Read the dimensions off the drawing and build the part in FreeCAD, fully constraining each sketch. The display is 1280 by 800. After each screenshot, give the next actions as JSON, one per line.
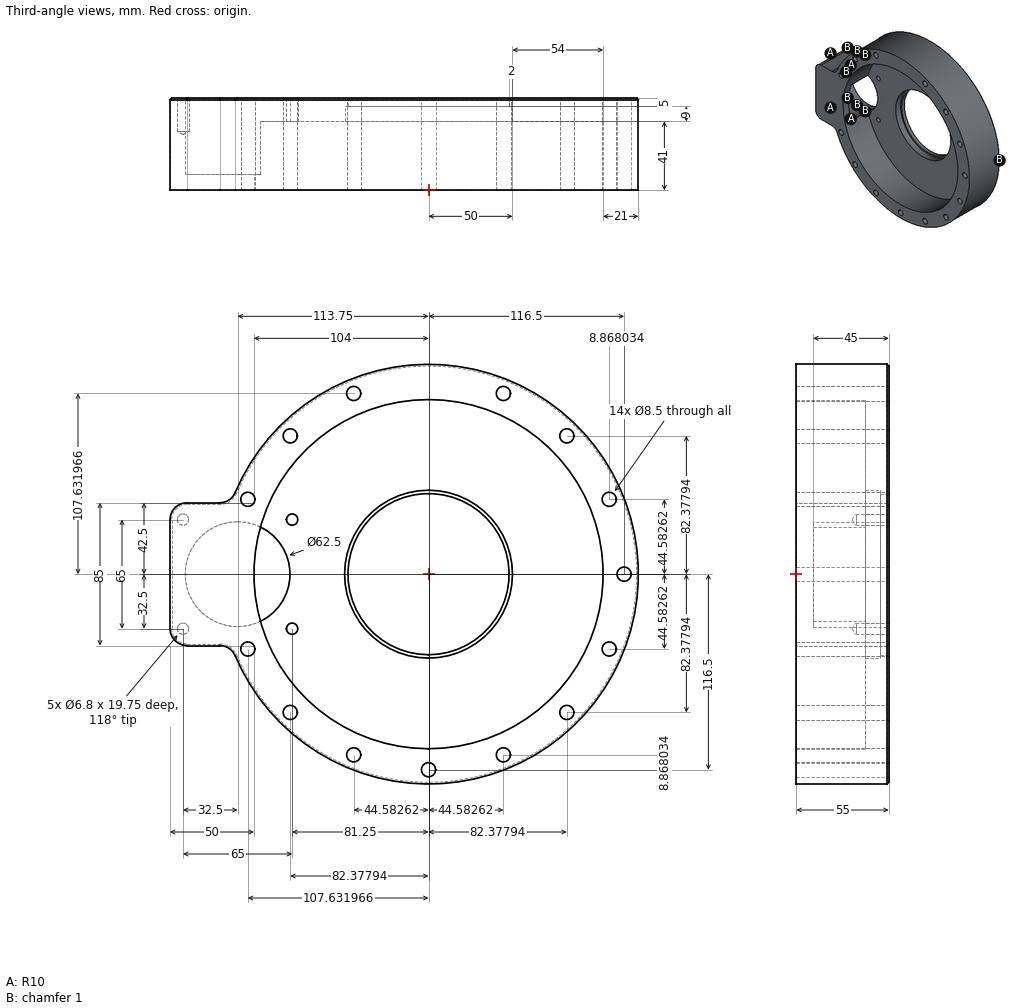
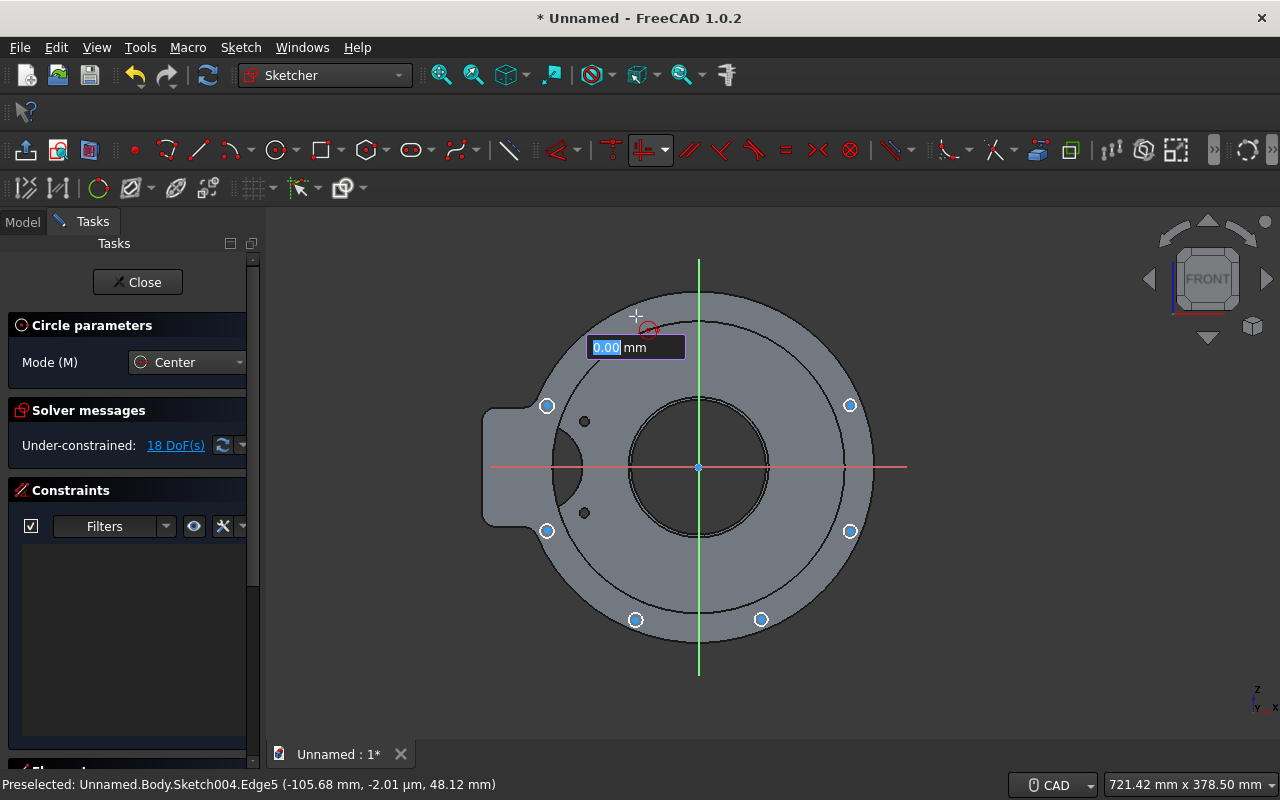
{"action": "scroll", "coordinate": [640, 312], "scroll_direction": "up", "scroll_amount": 5}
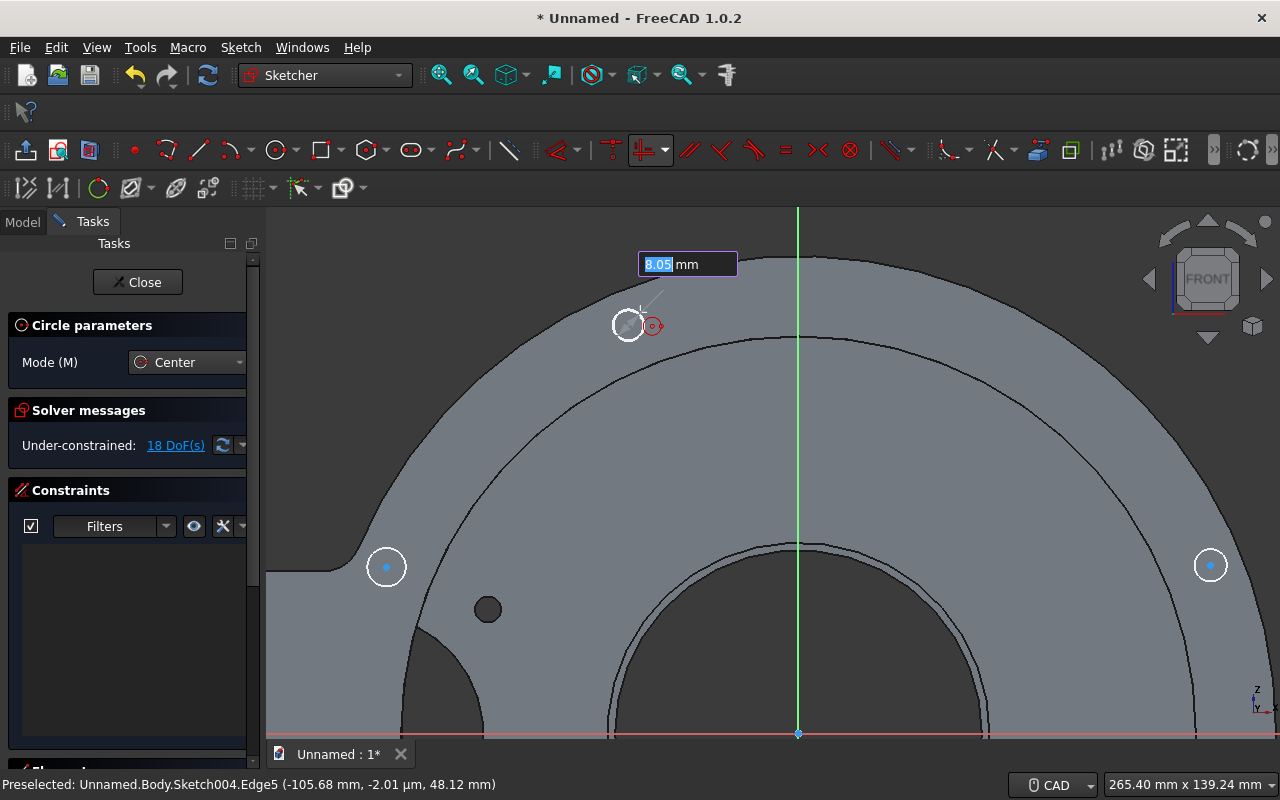
{"action": "left_click", "coordinate": [640, 311]}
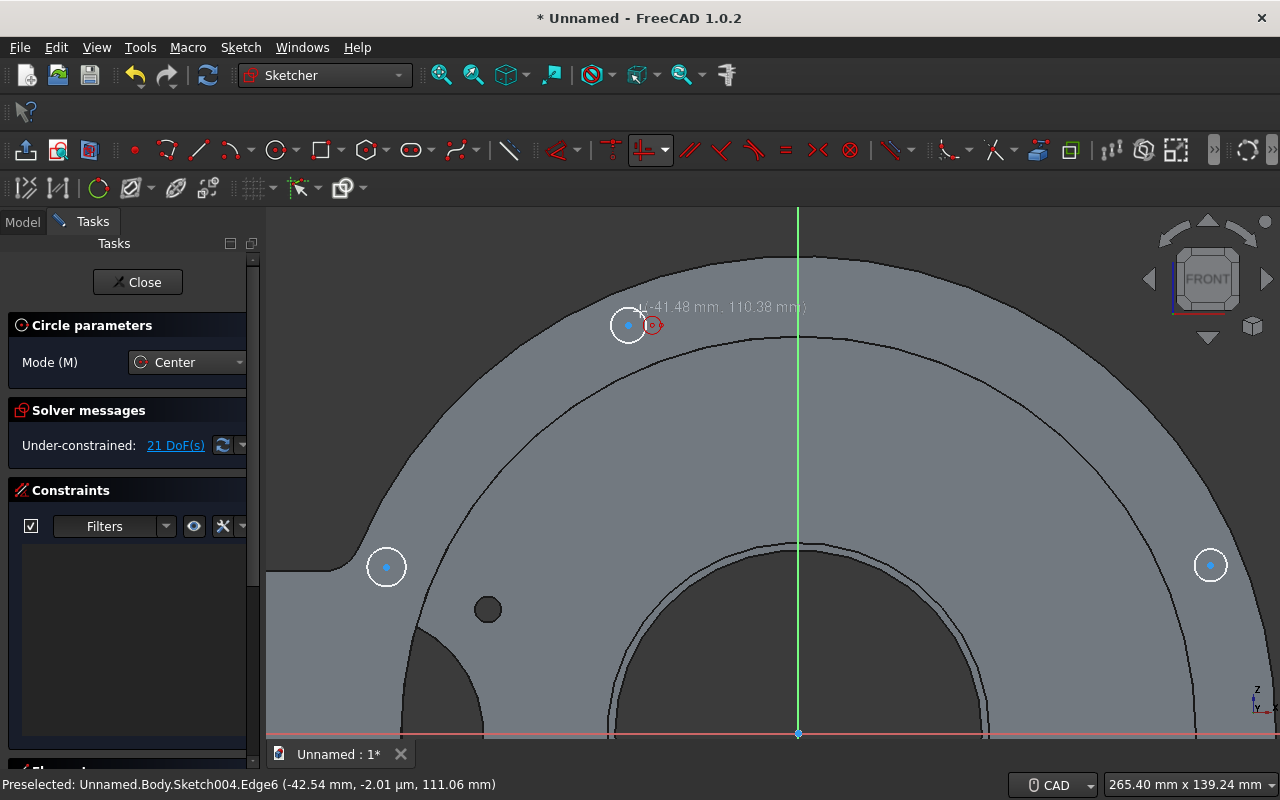
{"action": "scroll", "coordinate": [969, 323], "scroll_direction": "up", "scroll_amount": 2}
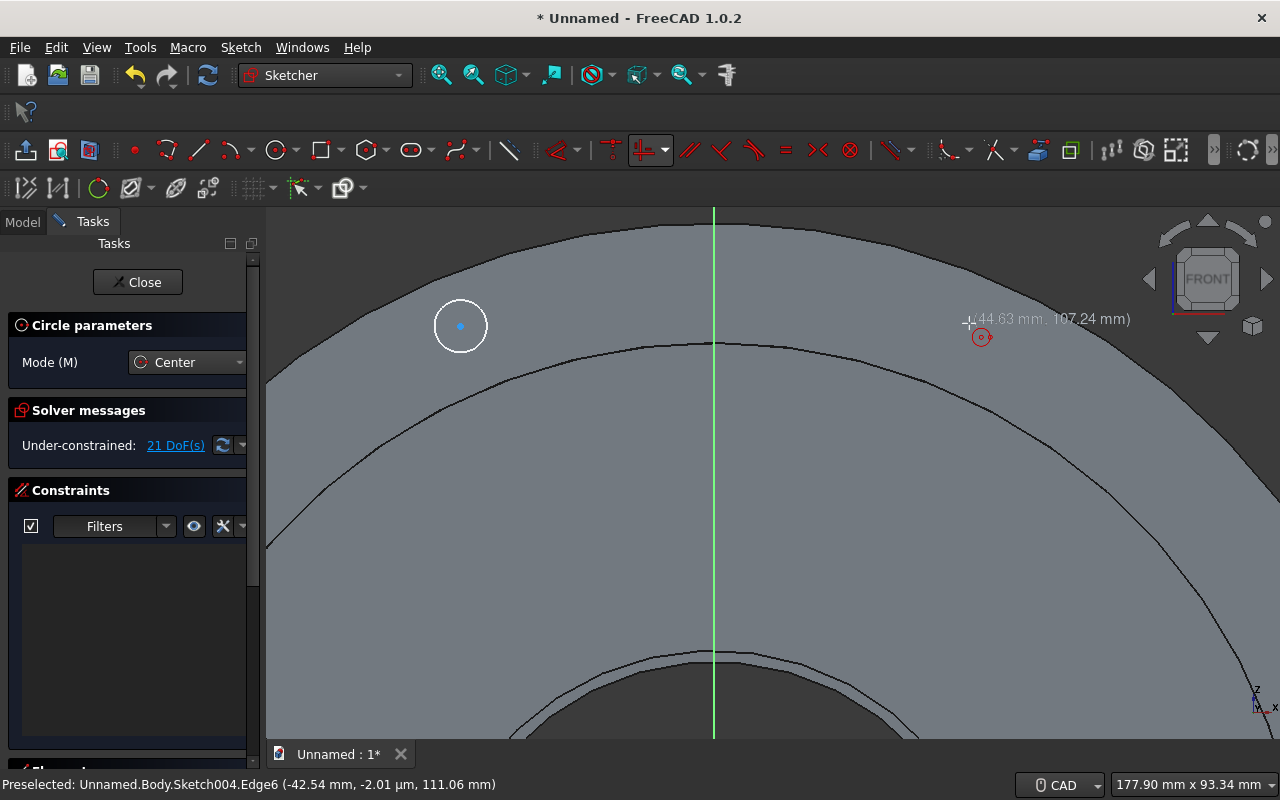
{"action": "scroll", "coordinate": [693, 313], "scroll_direction": "down", "scroll_amount": 7}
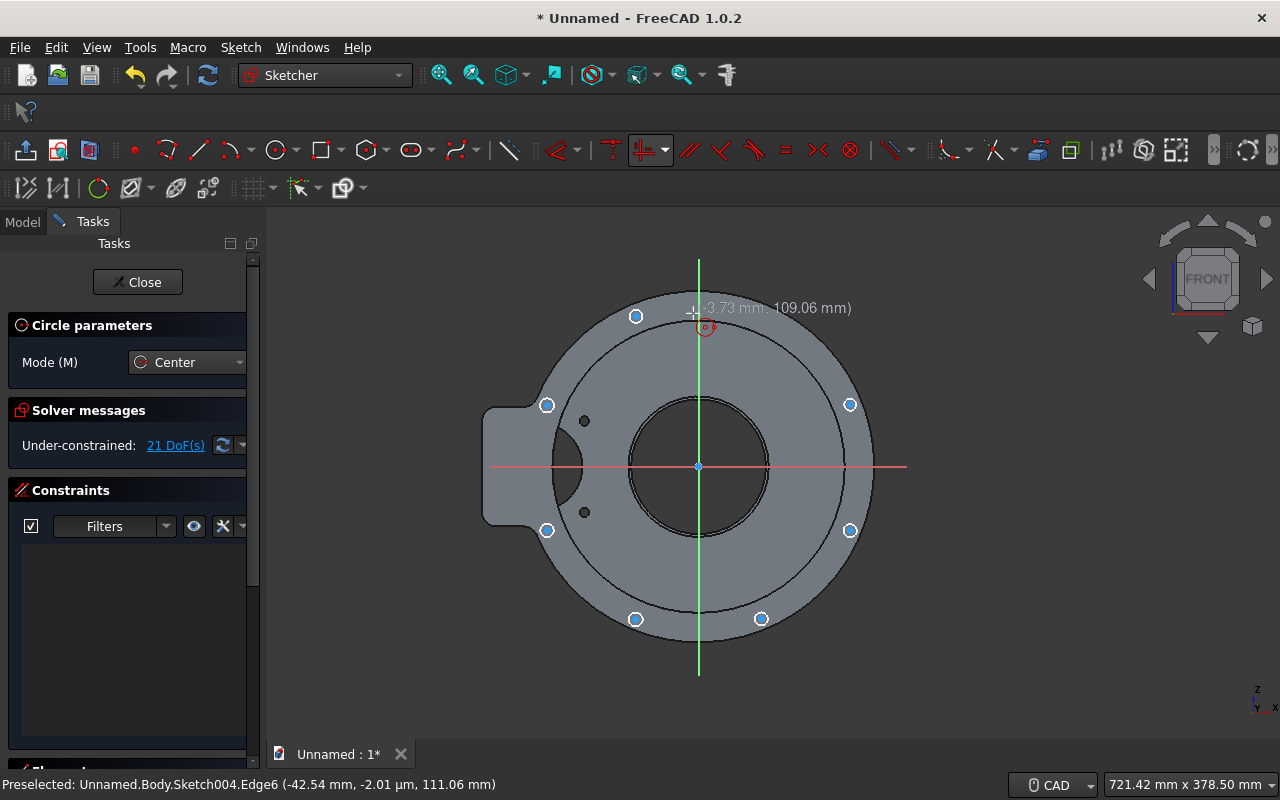
{"action": "left_click", "coordinate": [761, 315]}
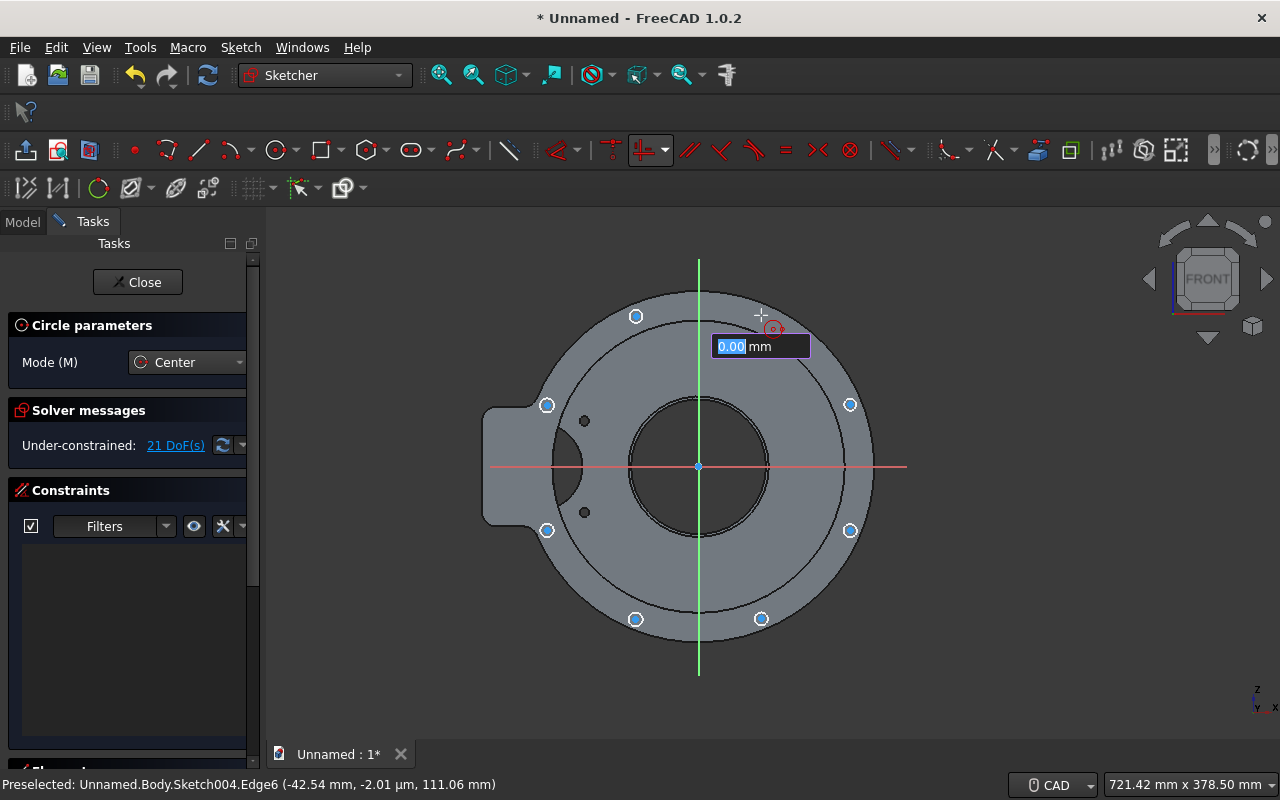
{"action": "scroll", "coordinate": [765, 311], "scroll_direction": "up", "scroll_amount": 5}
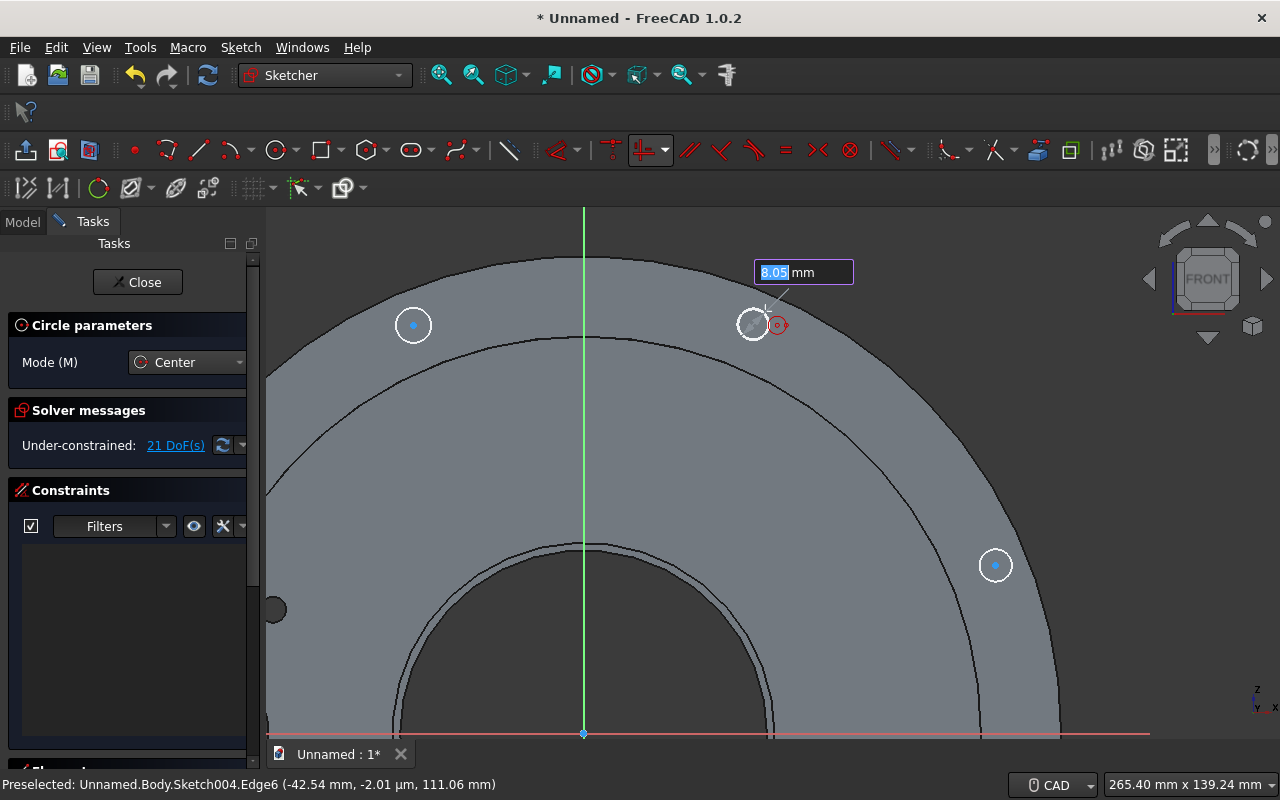
{"action": "left_click", "coordinate": [765, 311]}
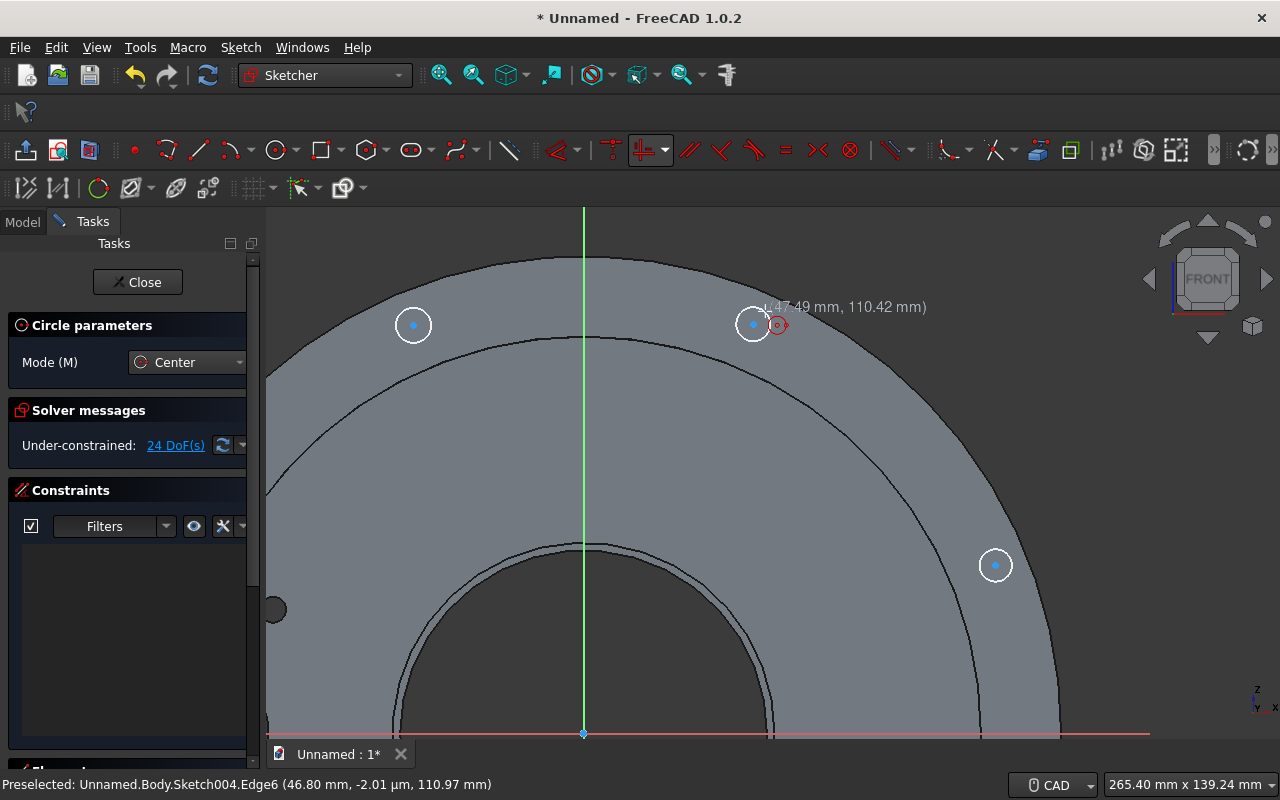
{"action": "scroll", "coordinate": [765, 311], "scroll_direction": "down", "scroll_amount": 5}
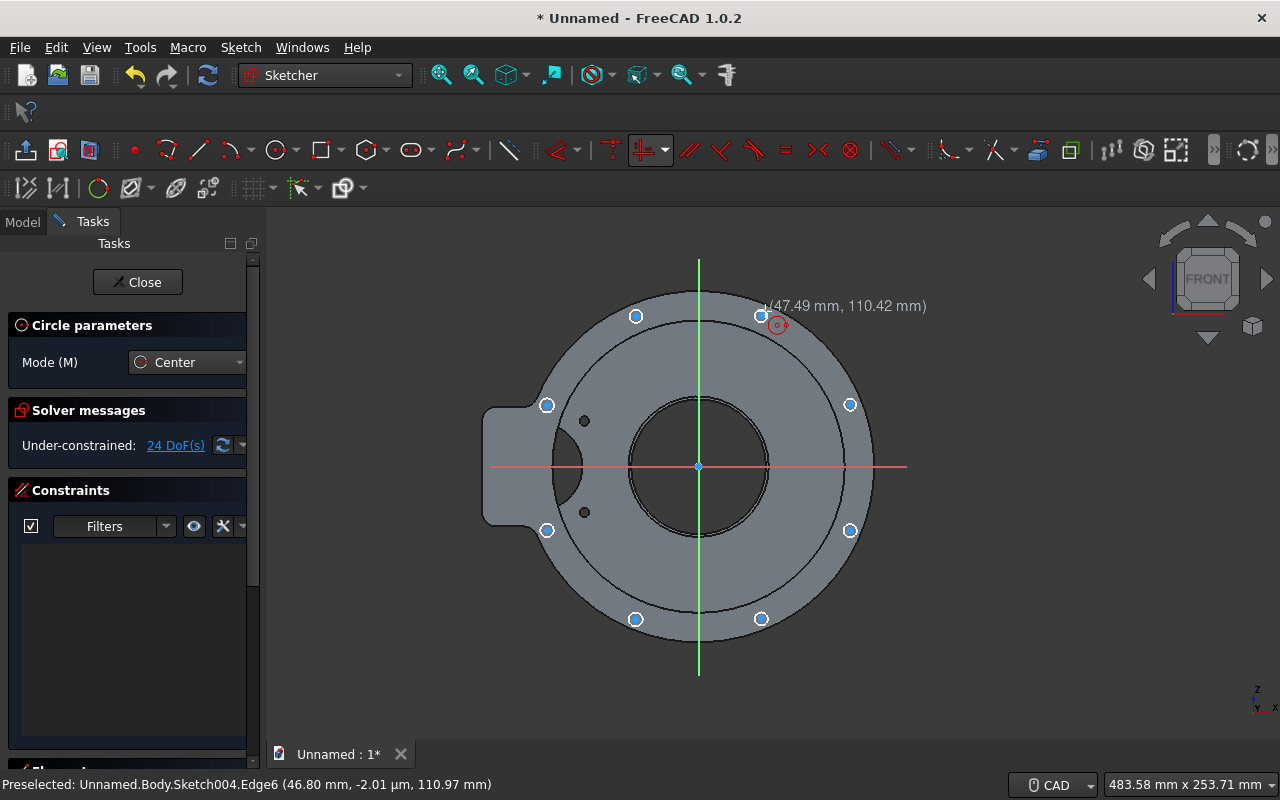
{"action": "scroll", "coordinate": [699, 630], "scroll_direction": "up", "scroll_amount": 7}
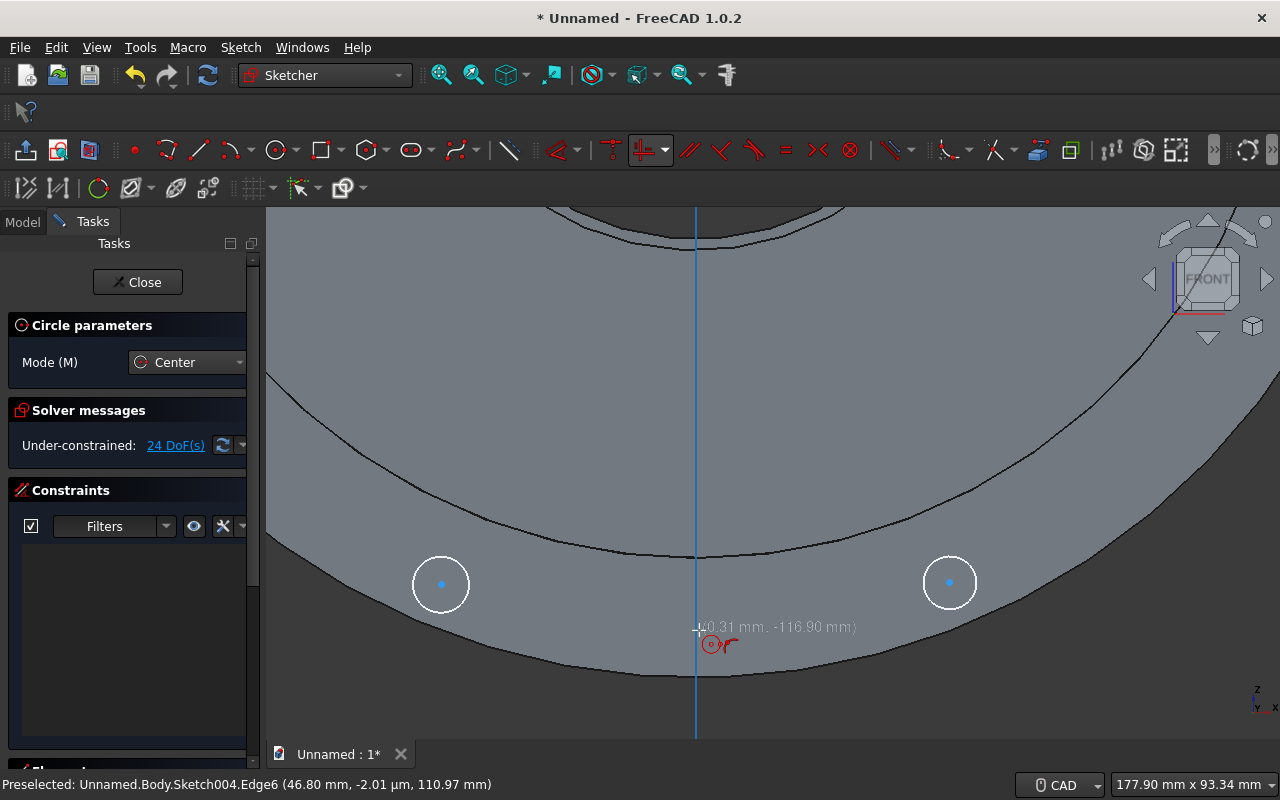
{"action": "scroll", "coordinate": [699, 631], "scroll_direction": "down", "scroll_amount": 7}